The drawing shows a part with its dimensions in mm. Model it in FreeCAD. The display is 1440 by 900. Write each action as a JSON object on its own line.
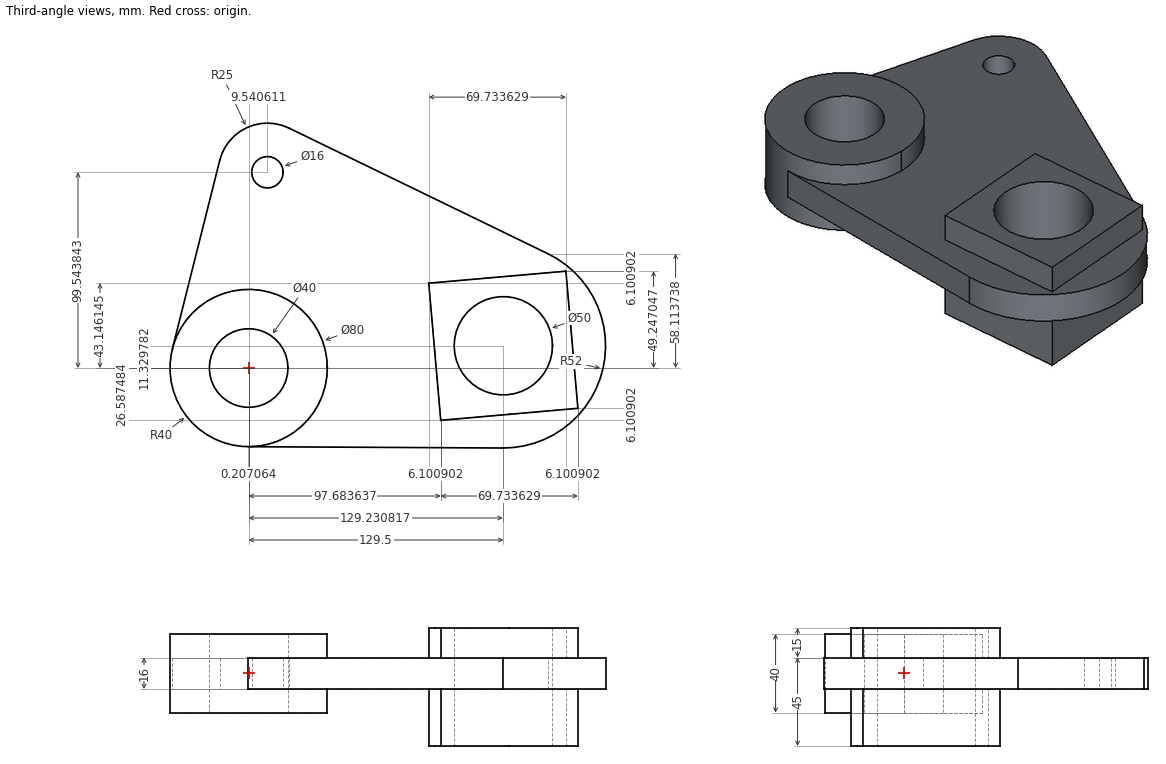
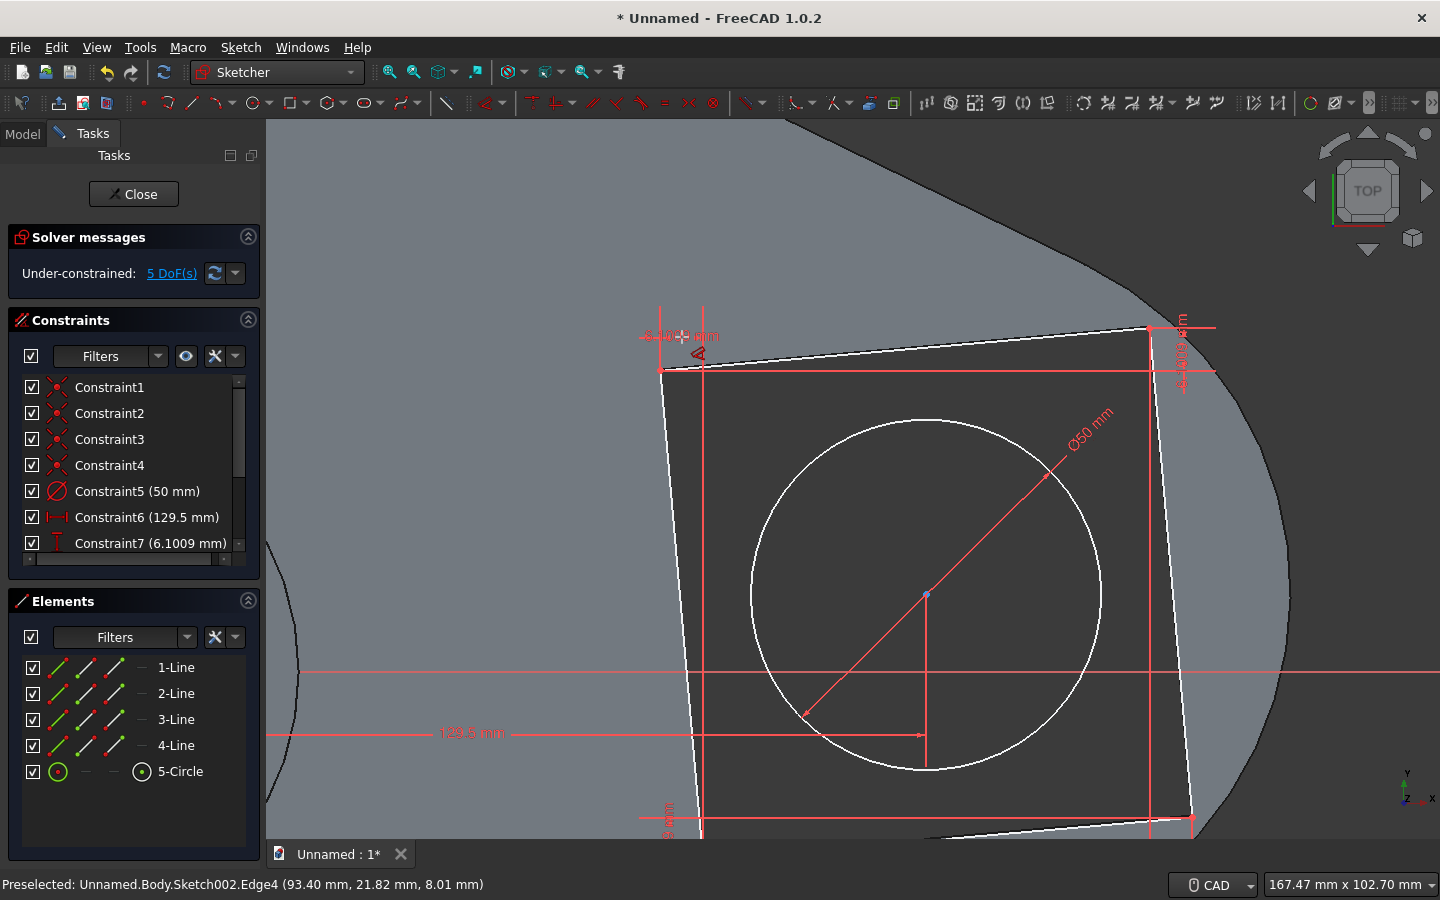
{"action": "left_click", "coordinate": [926, 595]}
{"action": "left_click", "coordinate": [960, 633]}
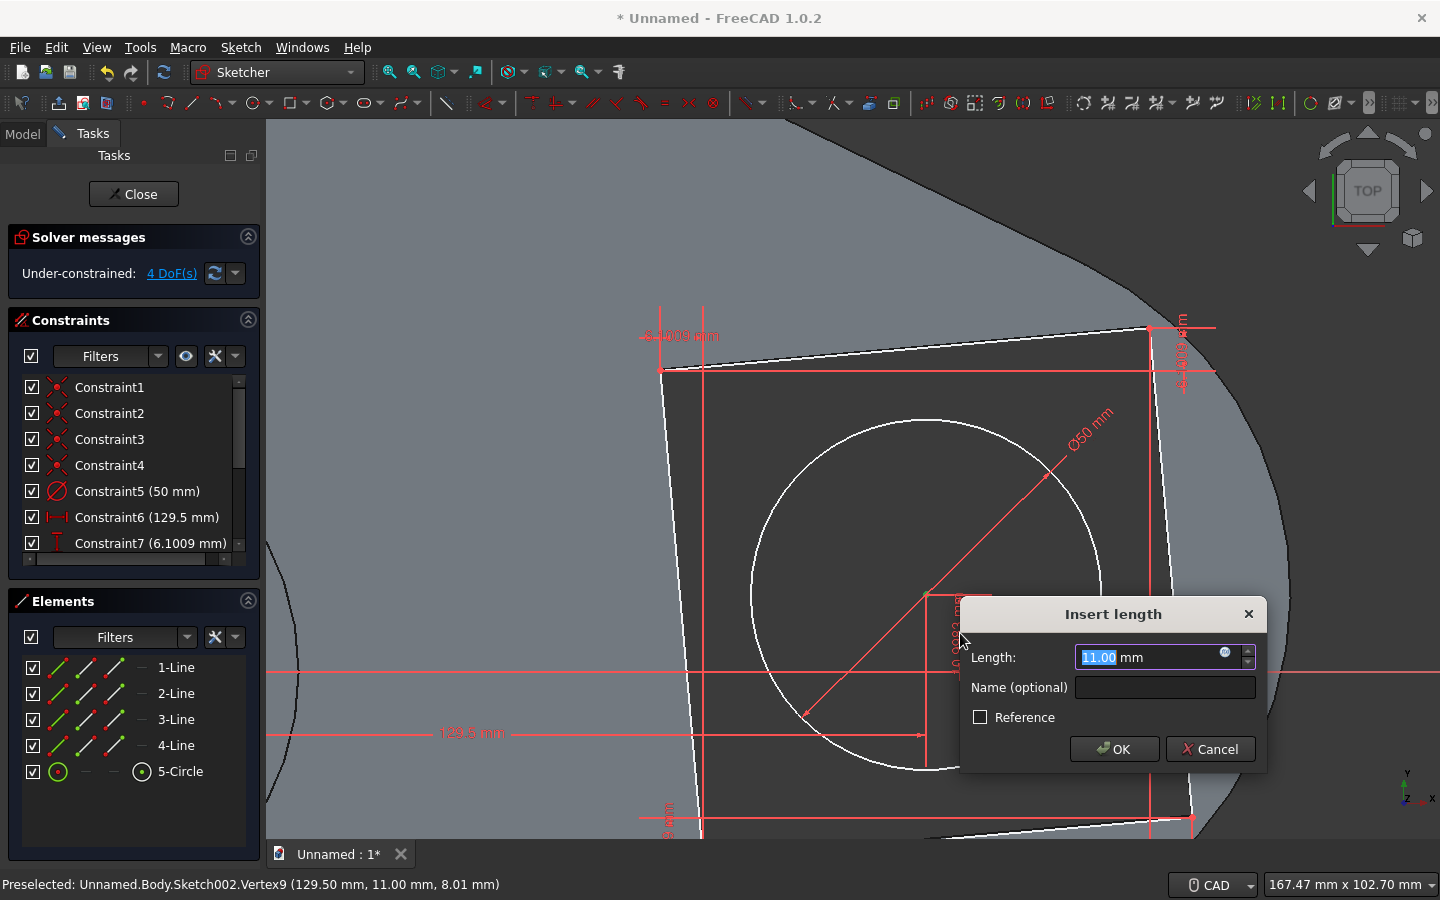
{"action": "type", "text": "11.329782"}
{"action": "key", "text": "Return"}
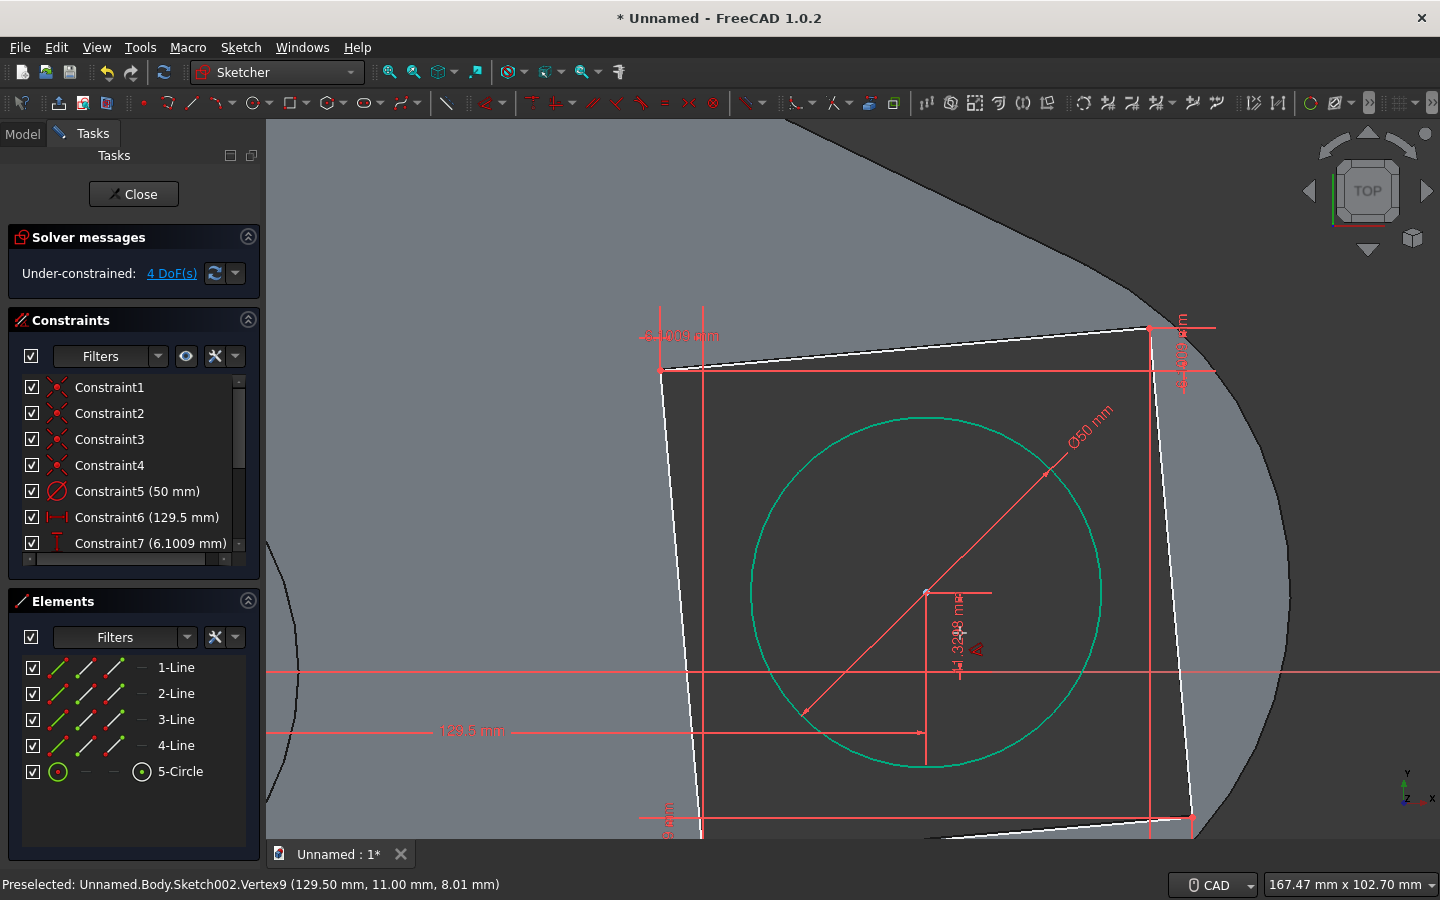
{"action": "scroll", "coordinate": [1003, 341], "scroll_direction": "down", "scroll_amount": 3}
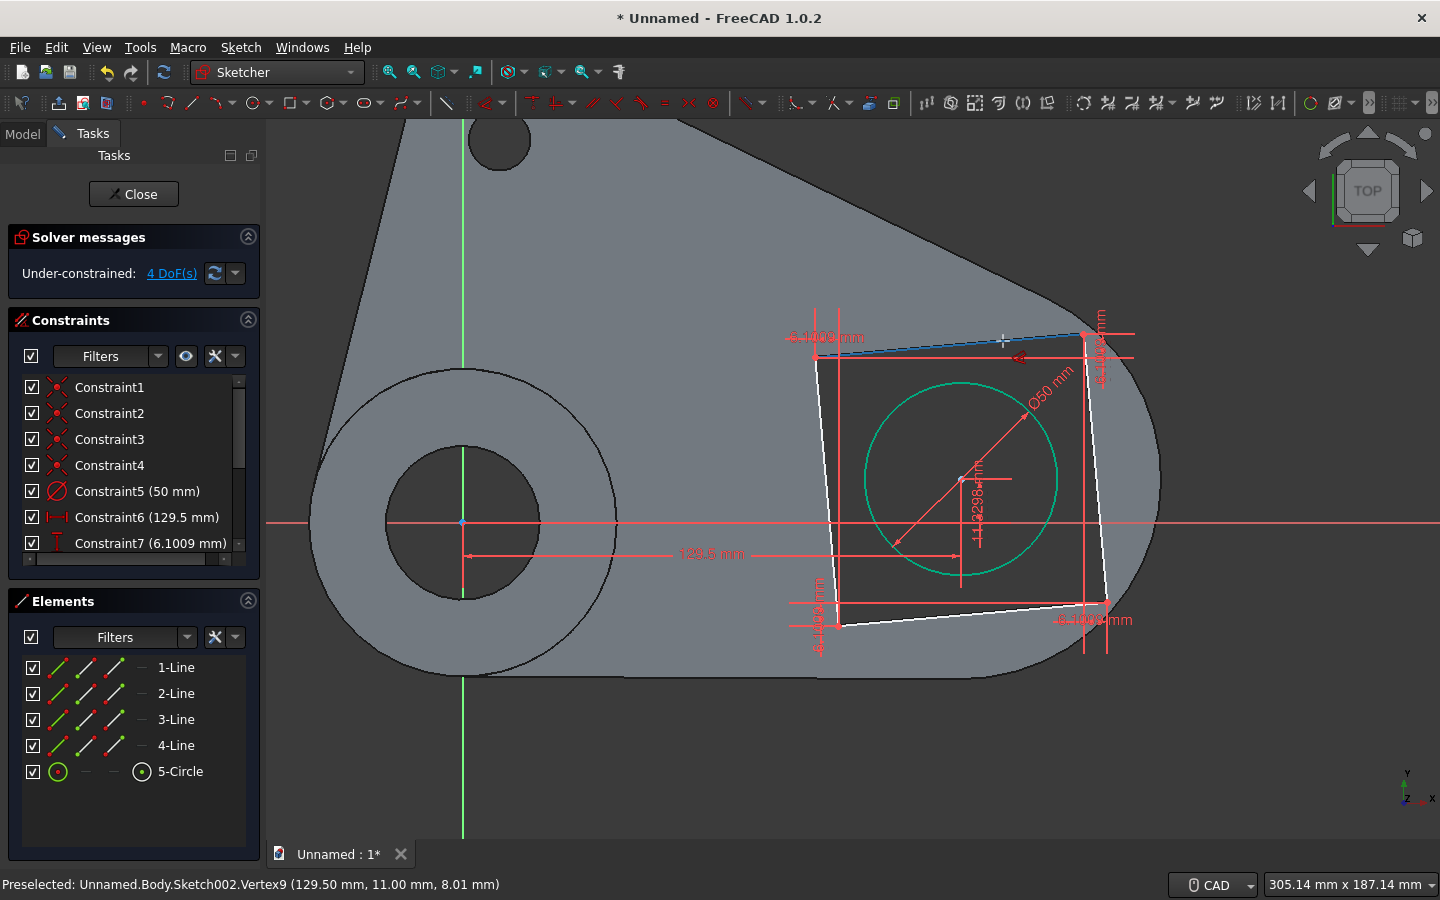
{"action": "left_click", "coordinate": [839, 626]}
{"action": "left_click", "coordinate": [651, 660]}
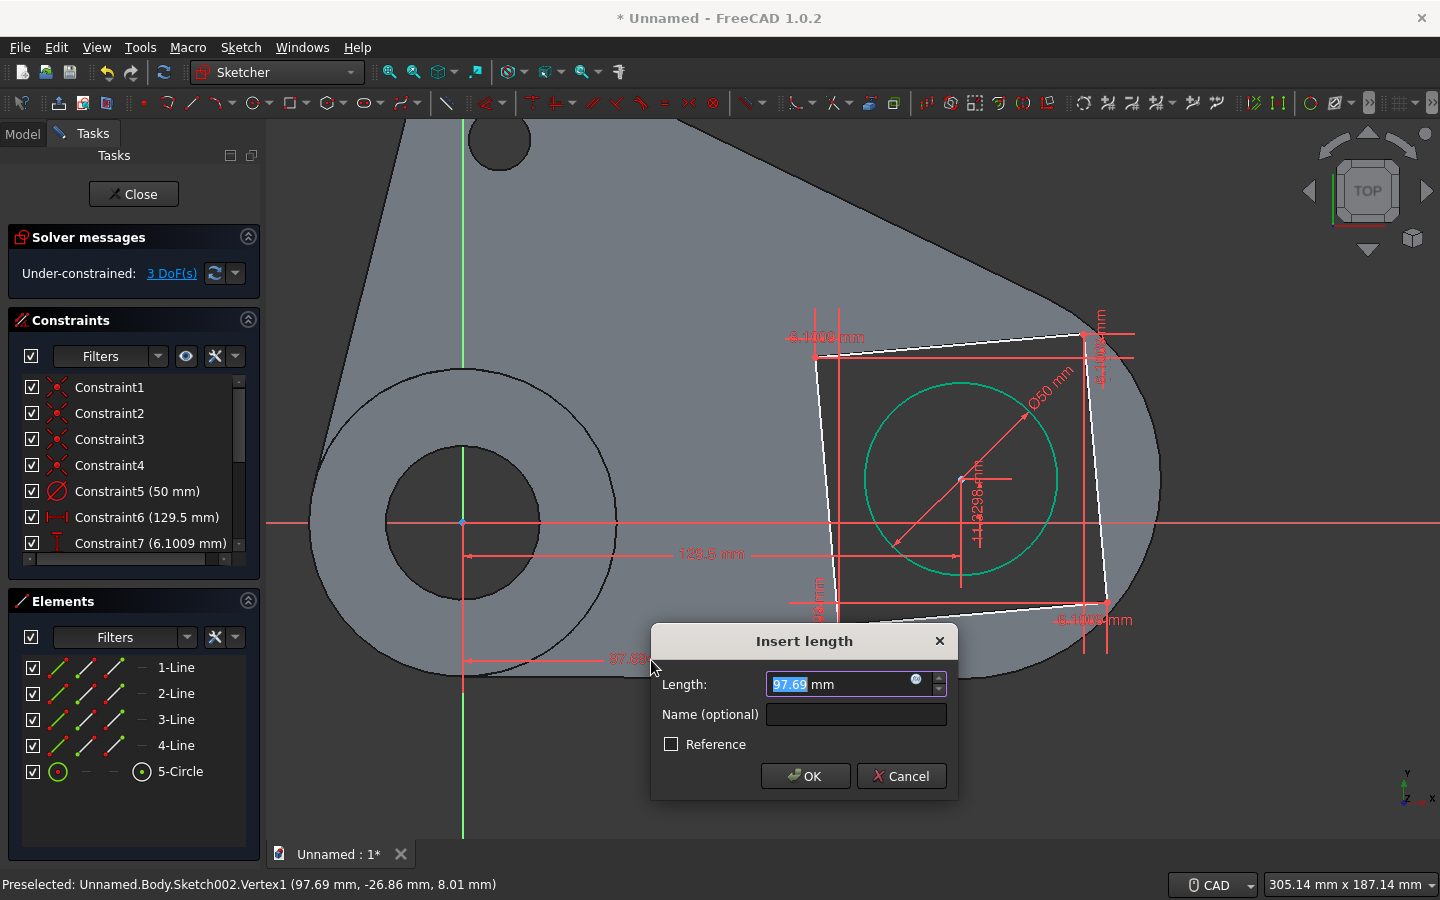
{"action": "type", "text": "97.683637"}
{"action": "key", "text": "Return"}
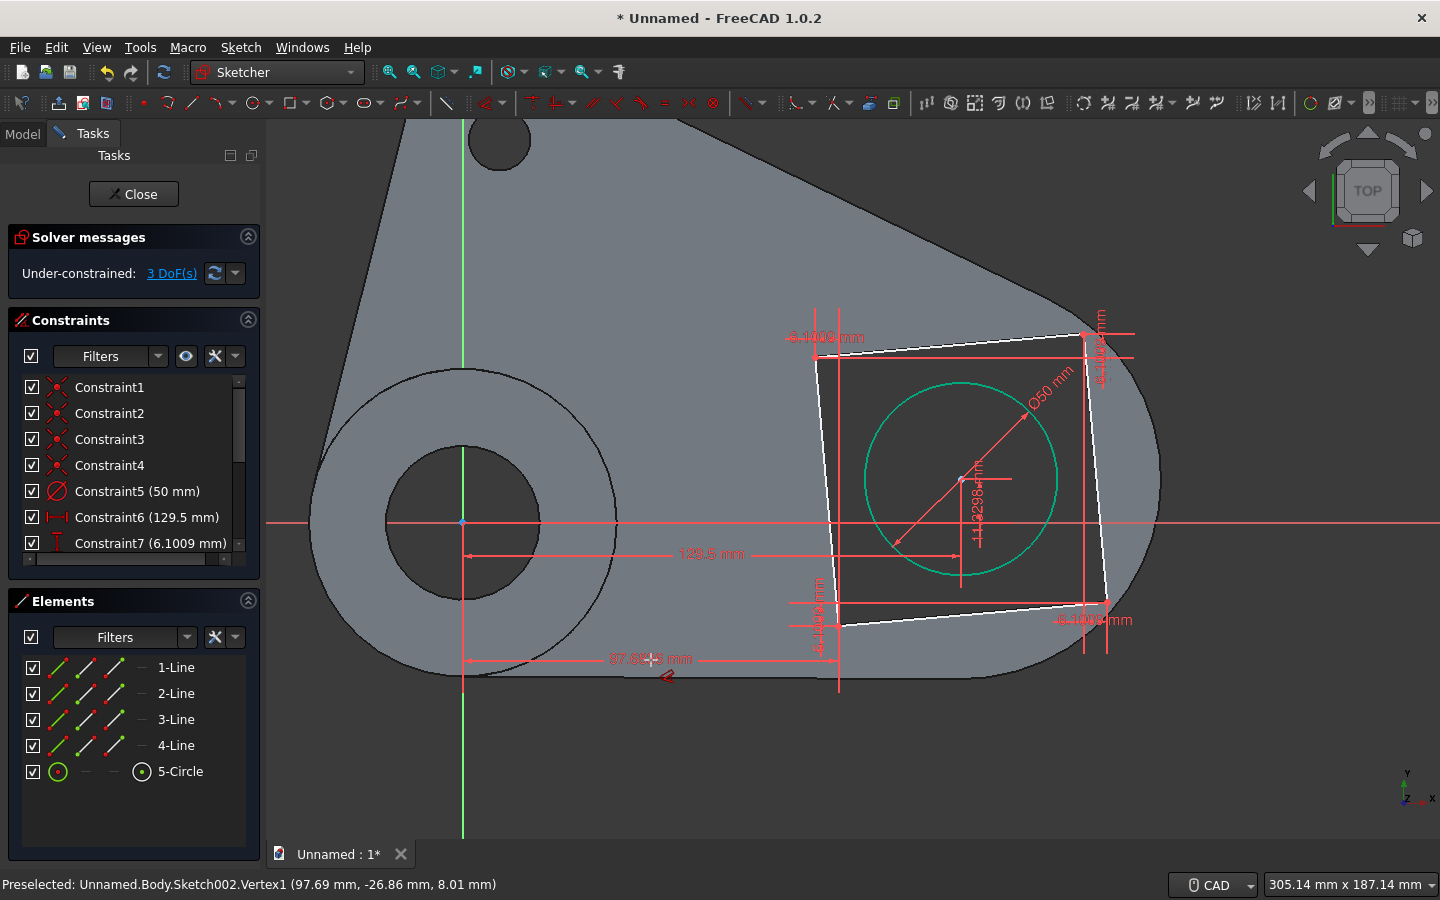
{"action": "left_click", "coordinate": [839, 626]}
{"action": "left_click", "coordinate": [429, 574]}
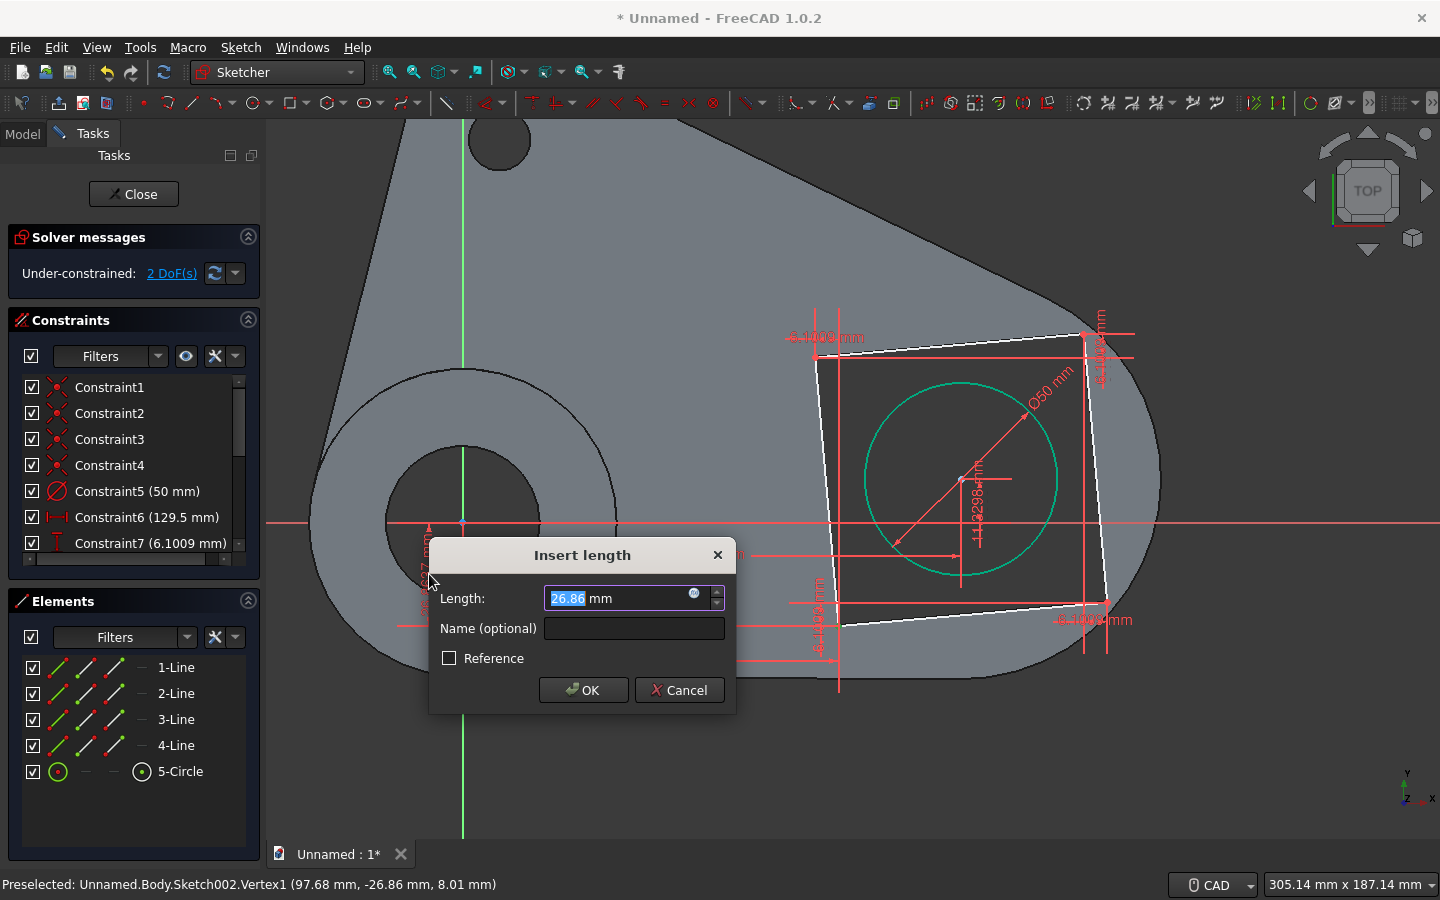
{"action": "type", "text": "26.587484"}
{"action": "key", "text": "Return"}